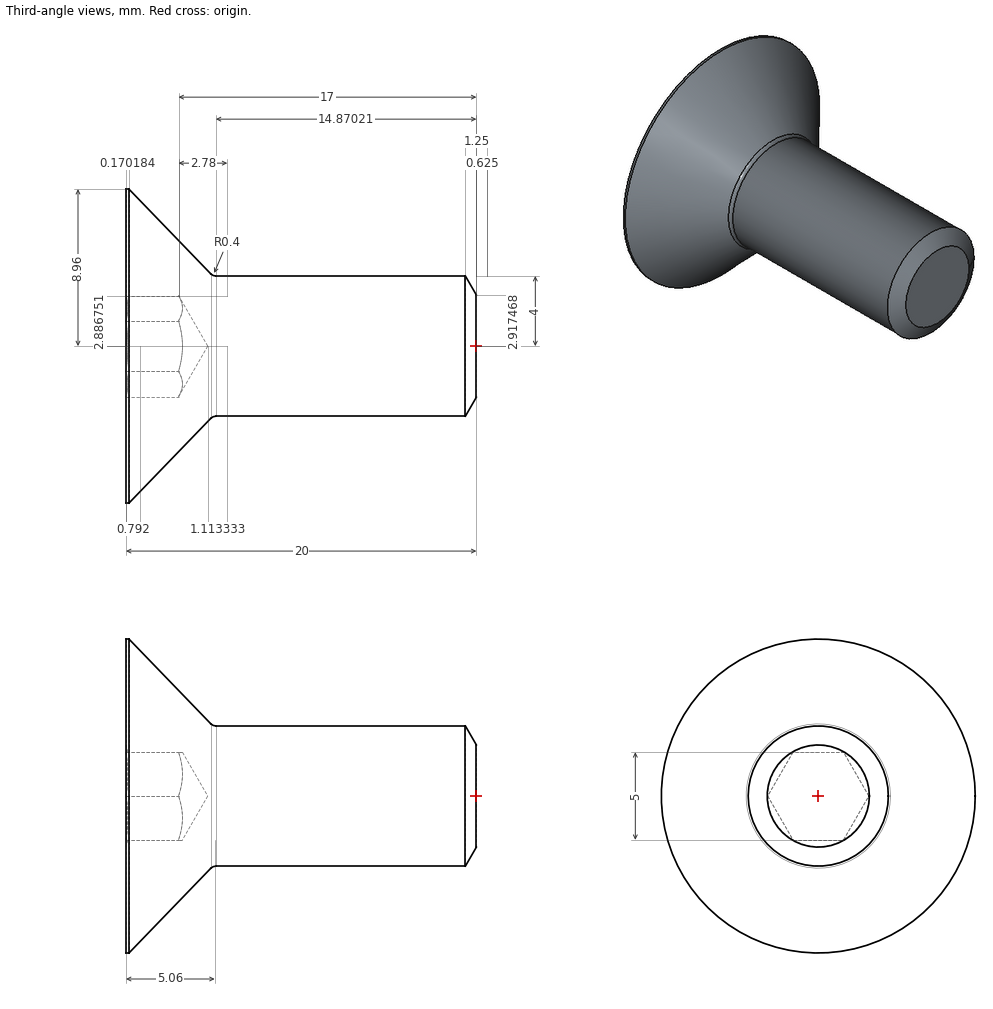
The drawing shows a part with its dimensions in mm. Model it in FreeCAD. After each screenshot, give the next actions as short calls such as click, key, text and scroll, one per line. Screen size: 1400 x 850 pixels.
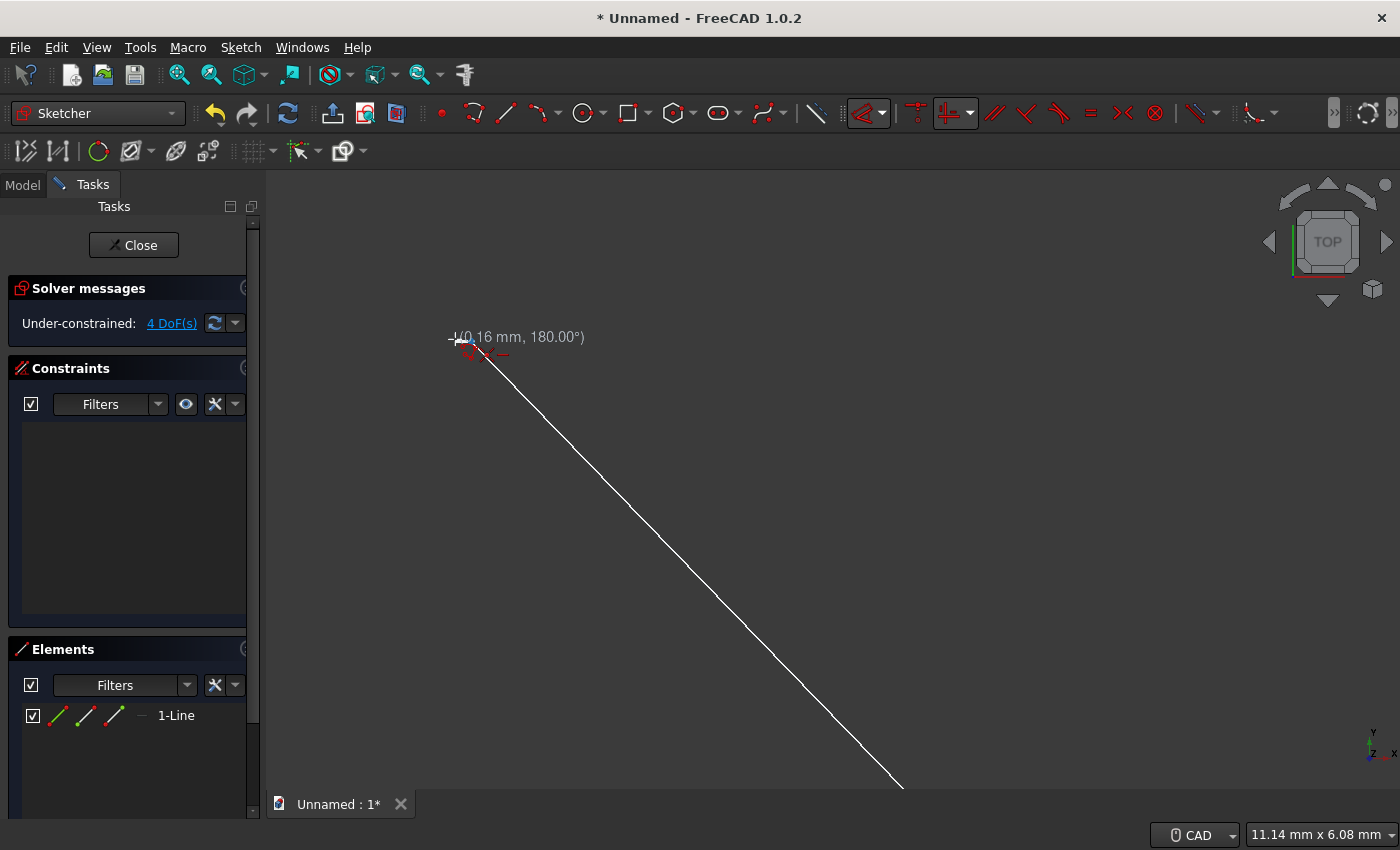
click(455, 338)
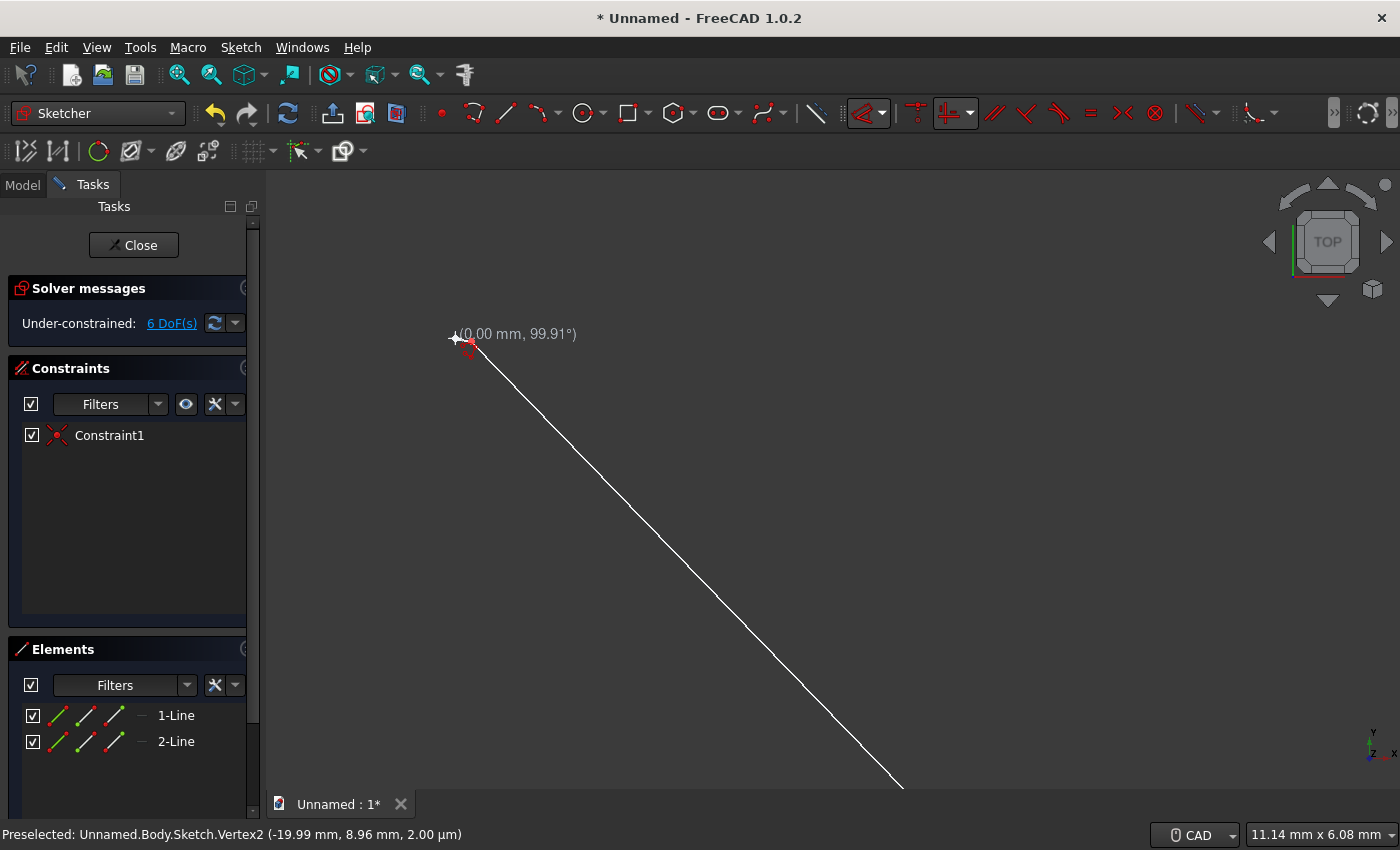
scroll(459, 343, down, 6)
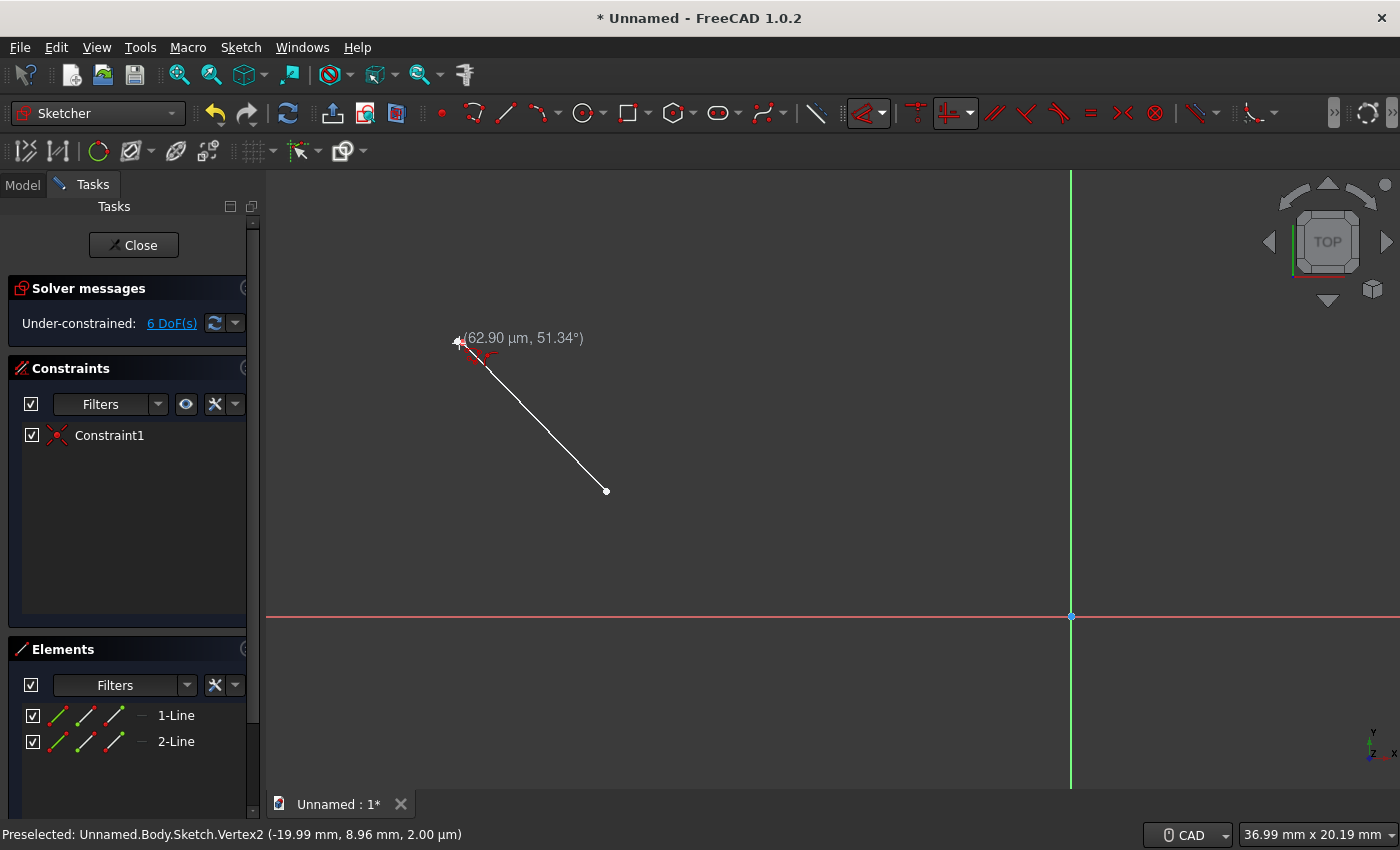
click(458, 617)
click(1071, 617)
click(1062, 494)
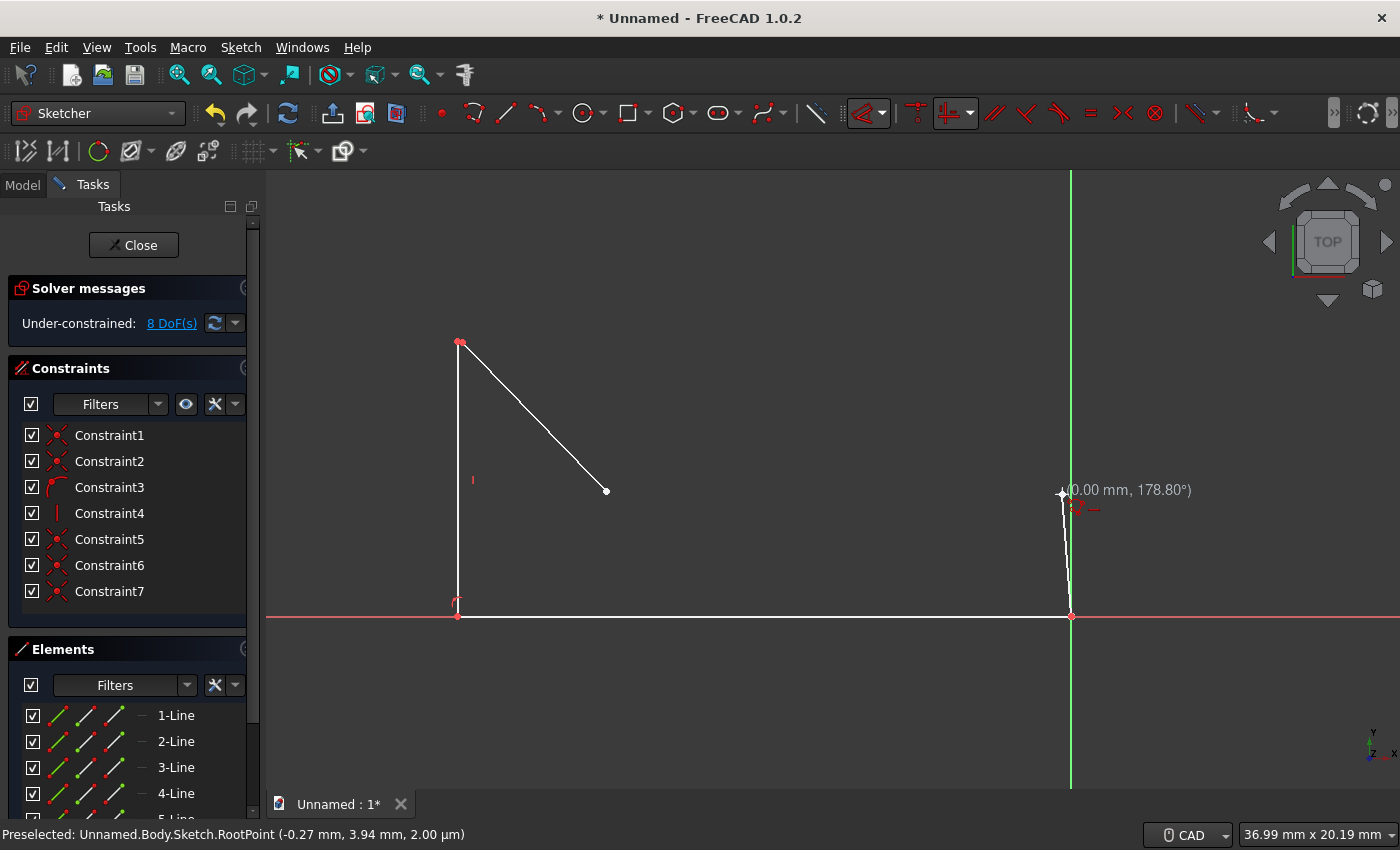
scroll(615, 494, up, 3)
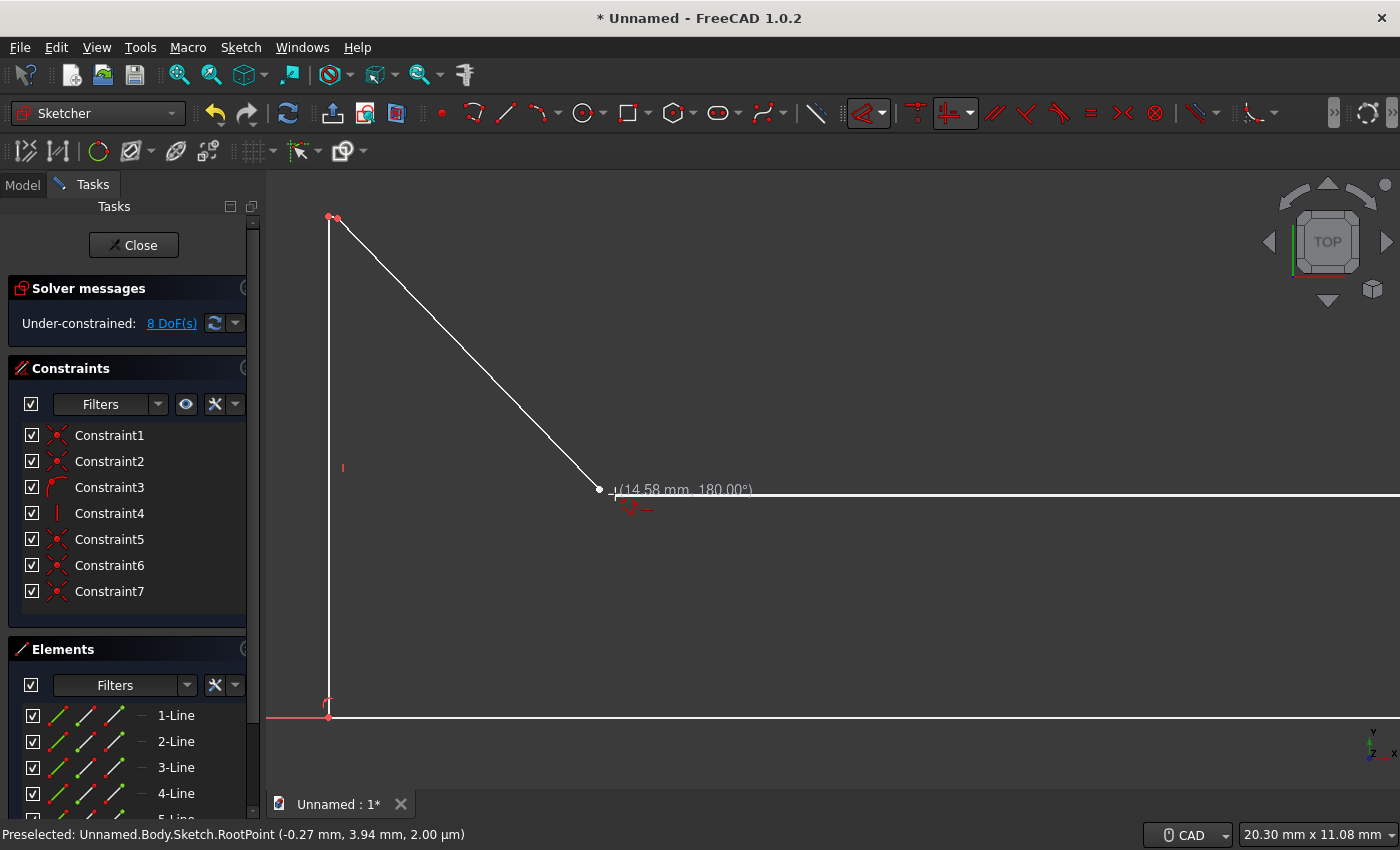
click(615, 494)
right_click(615, 494)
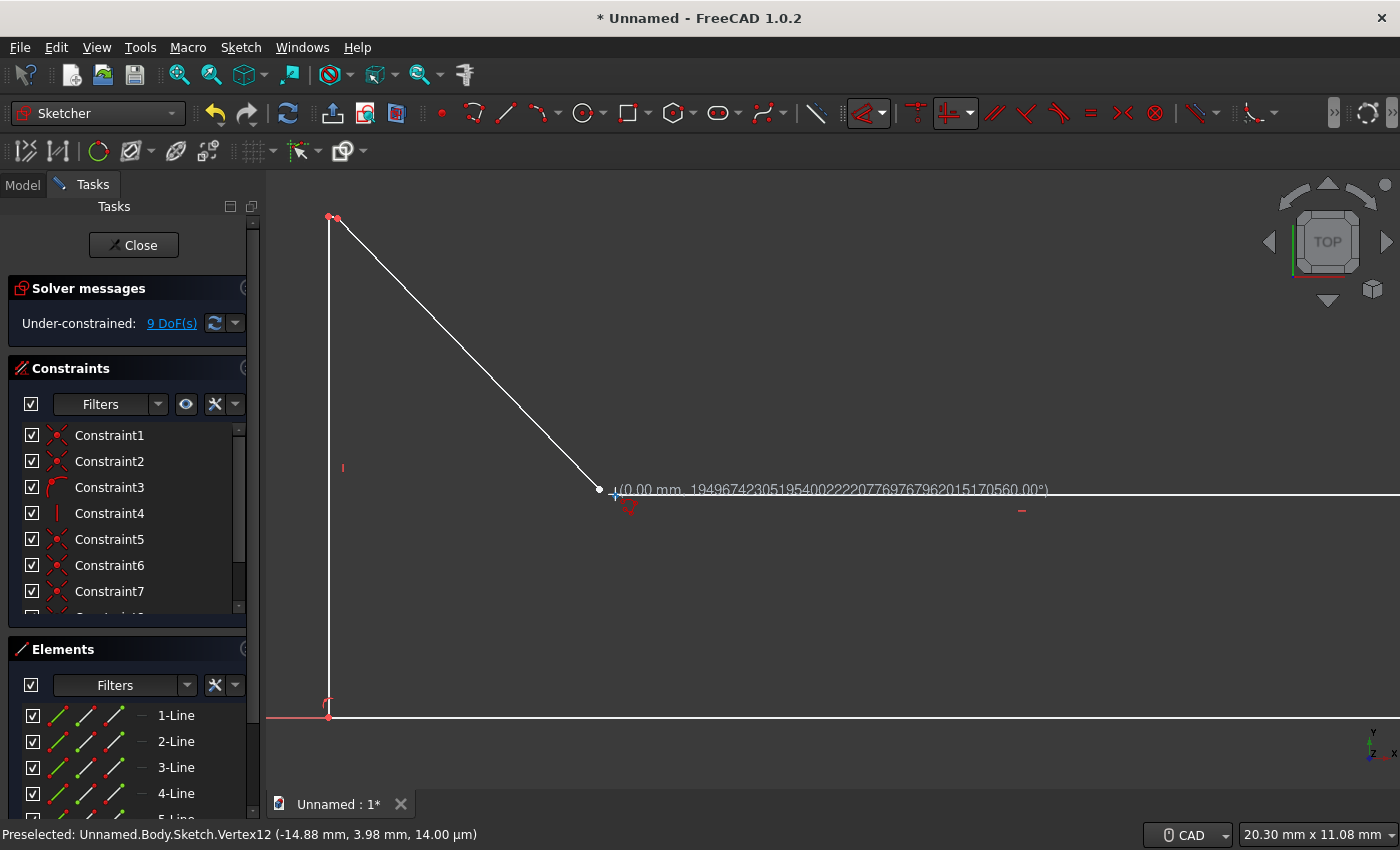
click(538, 114)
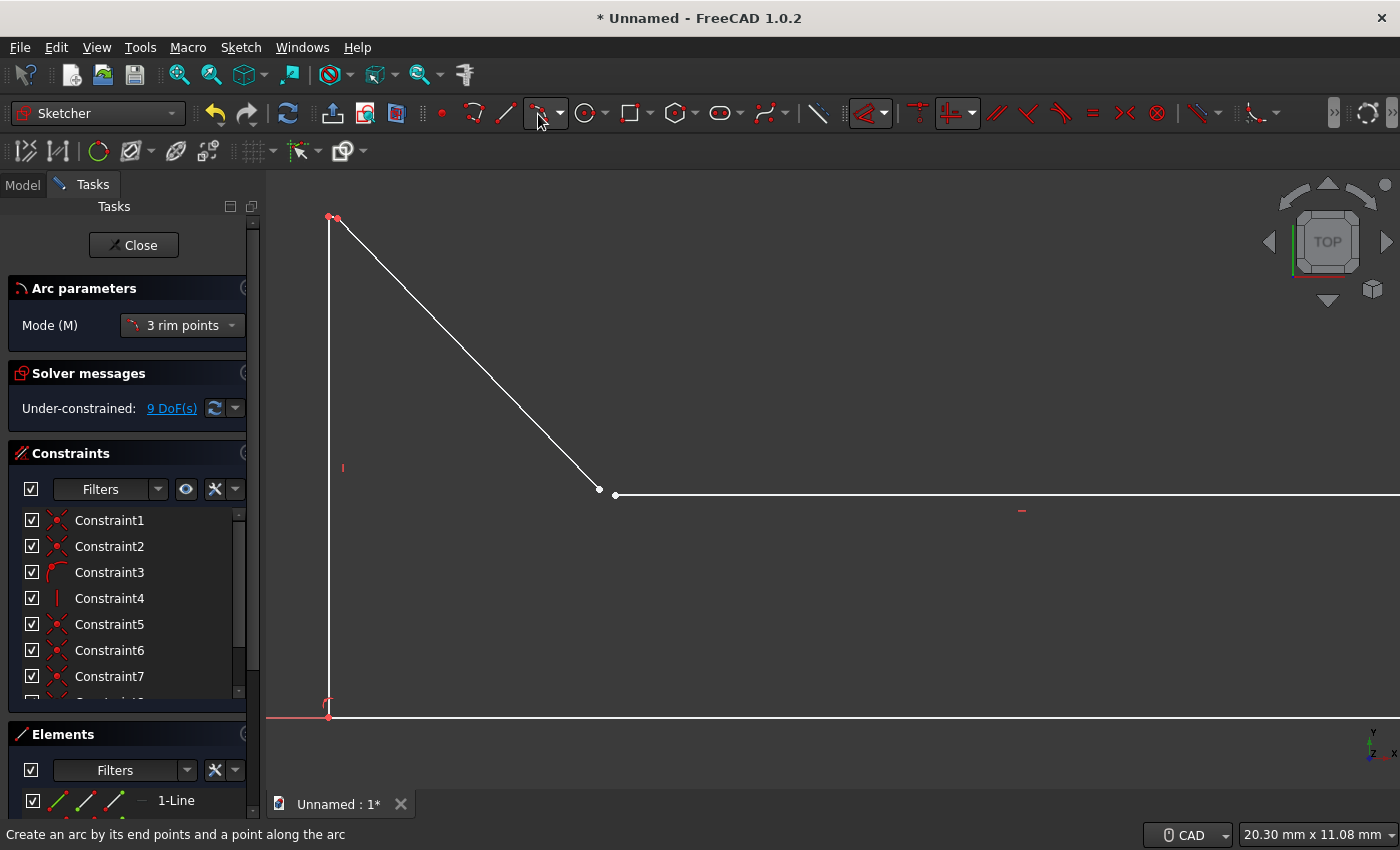
click(615, 495)
click(600, 490)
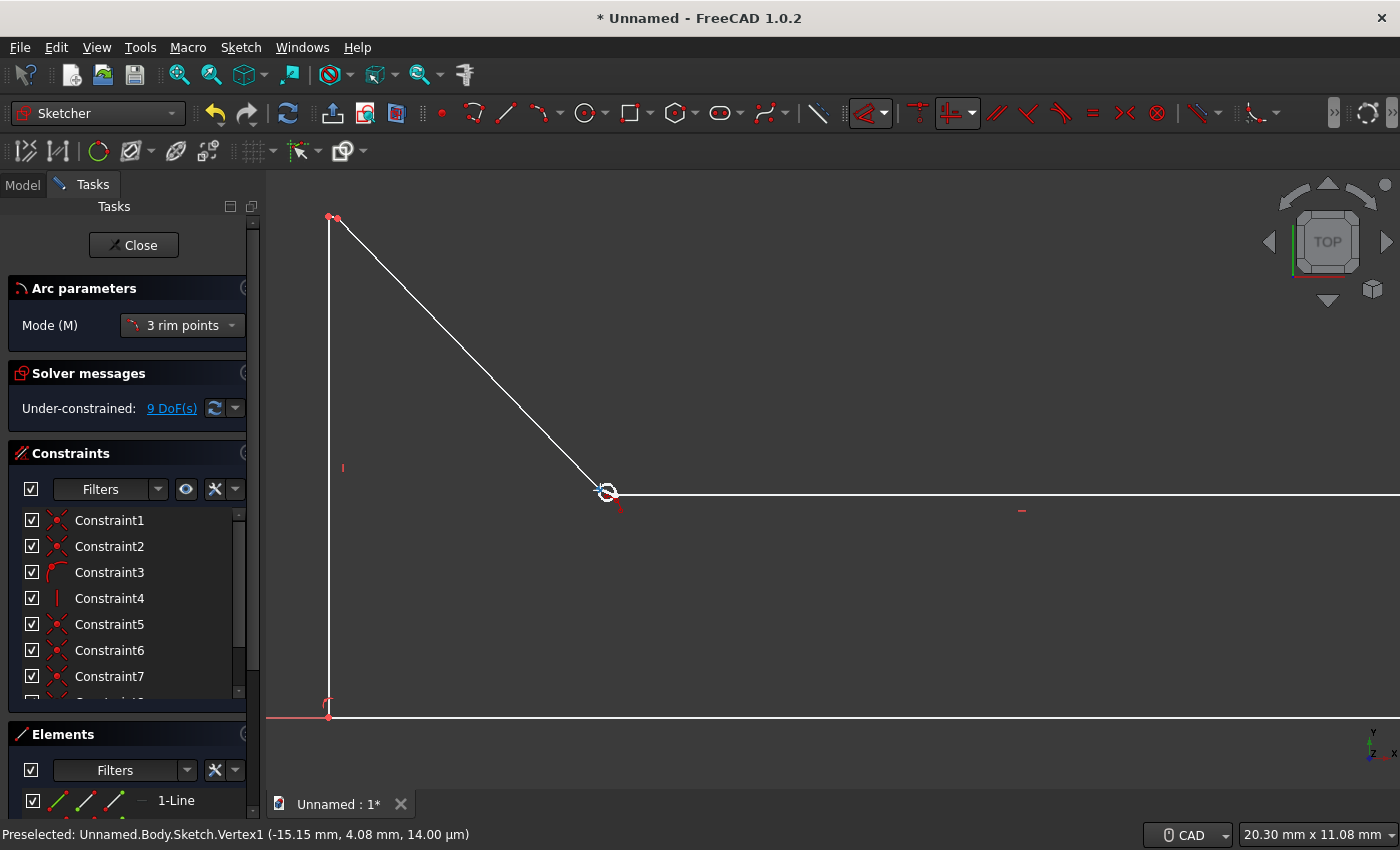
scroll(607, 492, up, 11)